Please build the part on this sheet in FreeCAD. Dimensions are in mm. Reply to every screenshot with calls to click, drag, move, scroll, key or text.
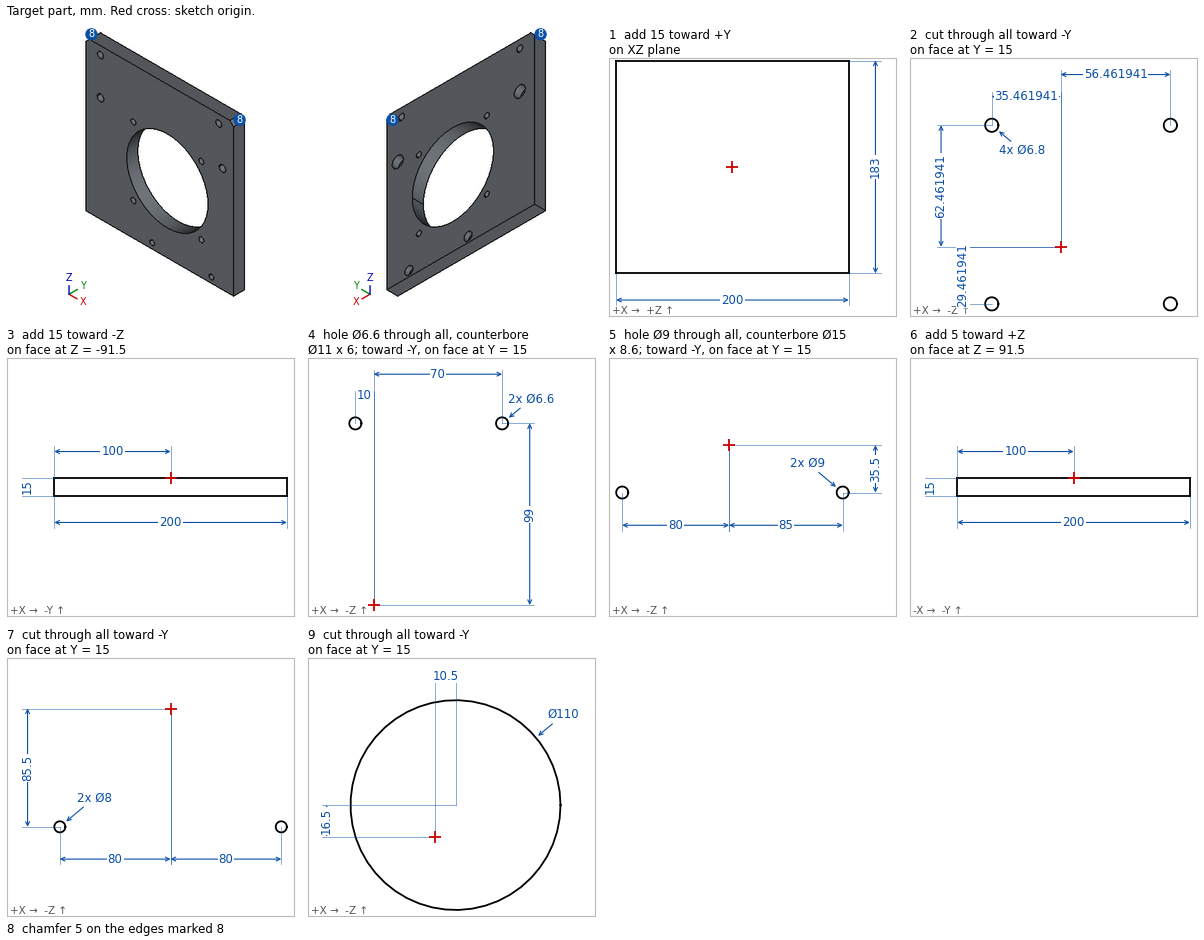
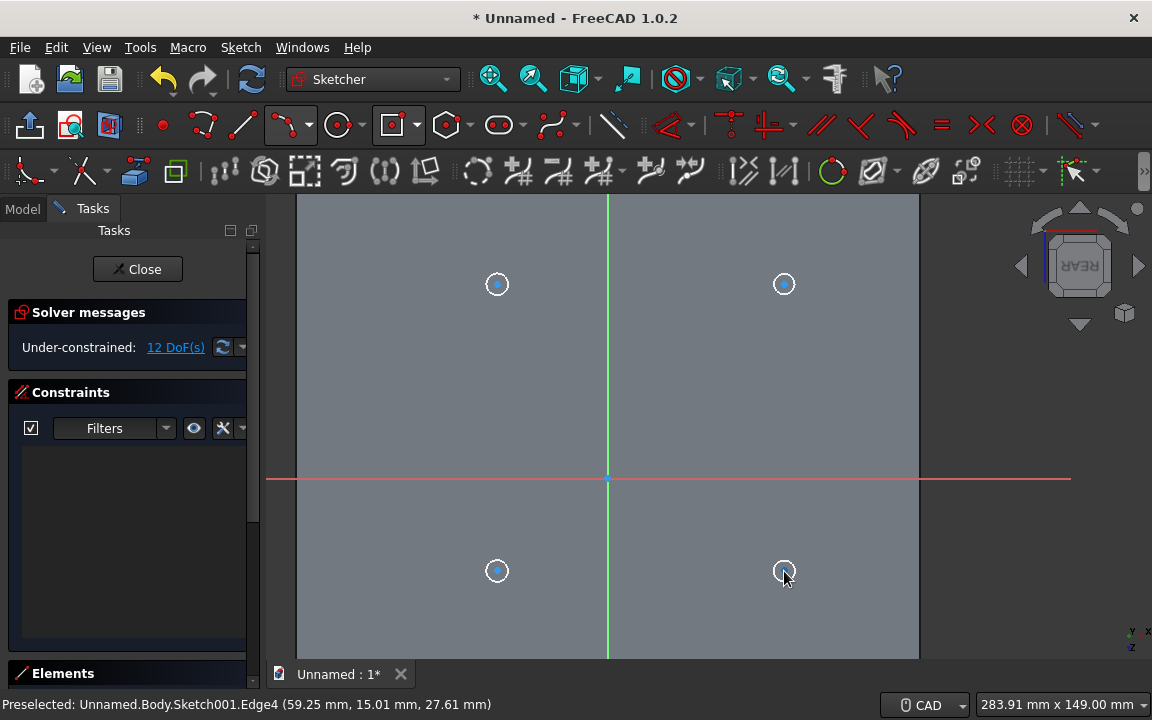
scroll(505, 277, up, 2)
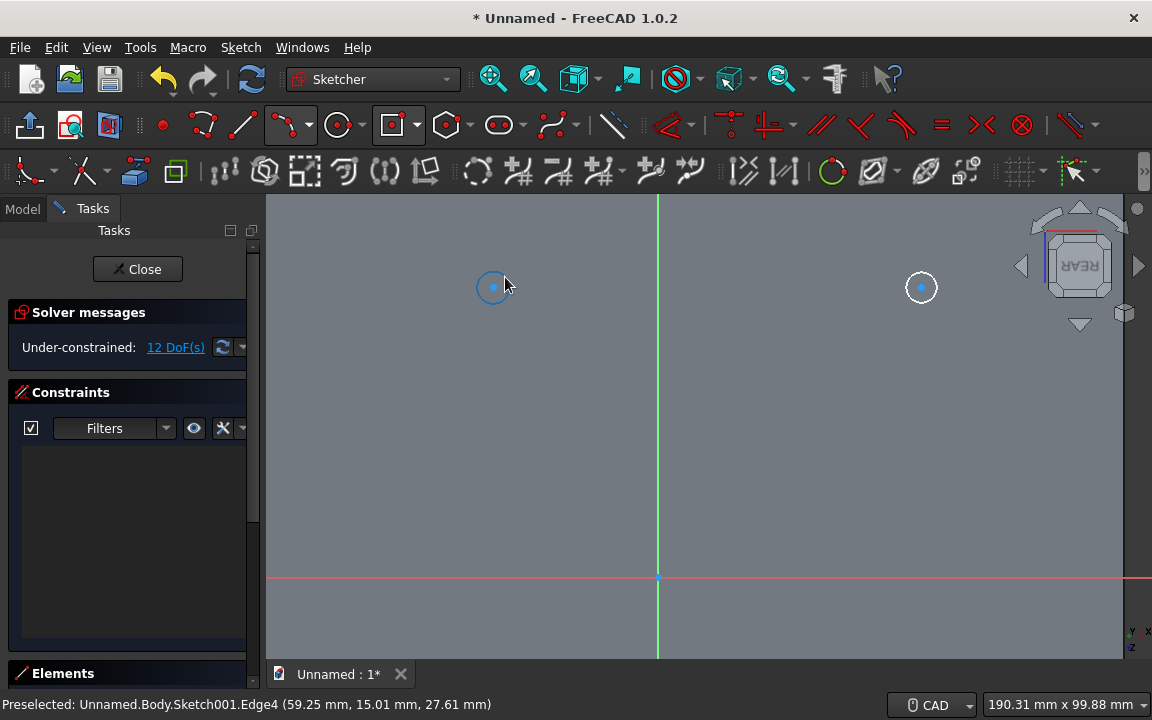
click(505, 276)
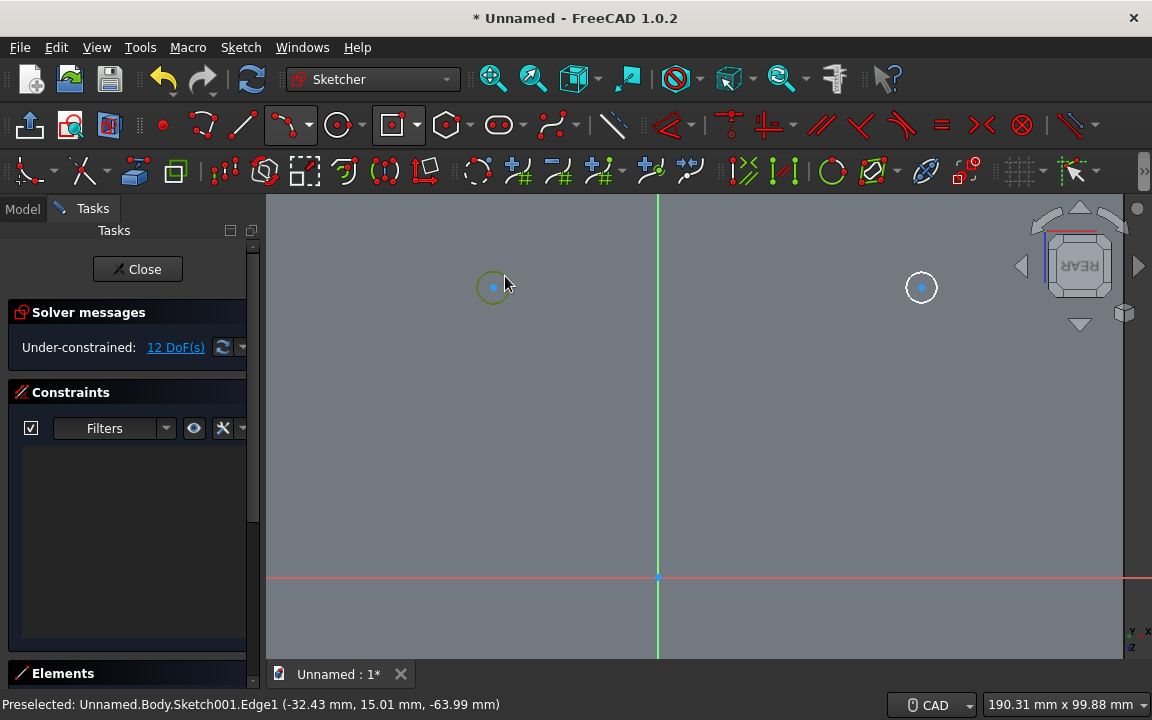
click(932, 277)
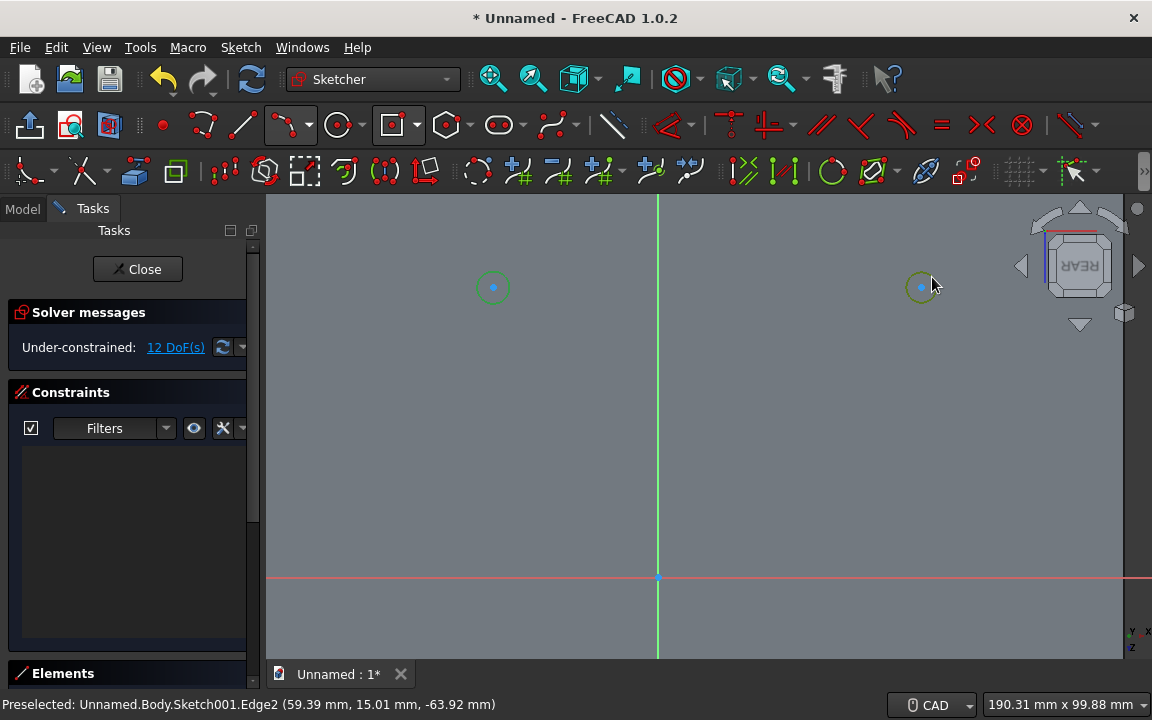
scroll(505, 275, down, 2)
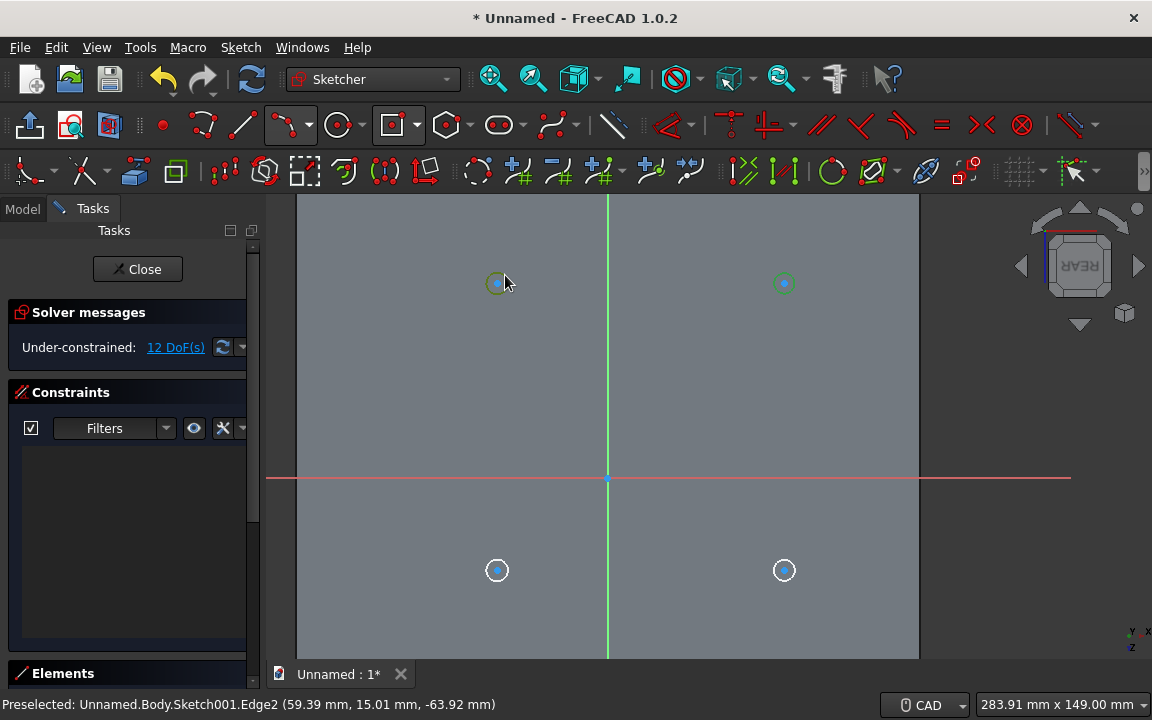
scroll(505, 563, up, 2)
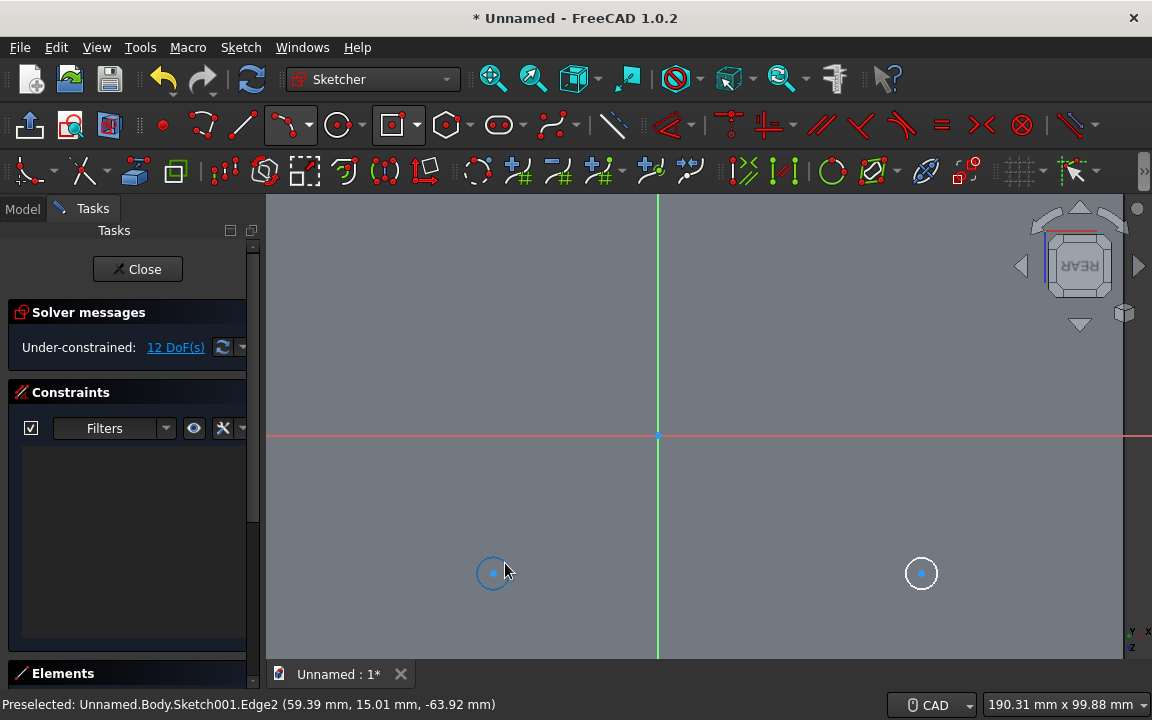
click(505, 562)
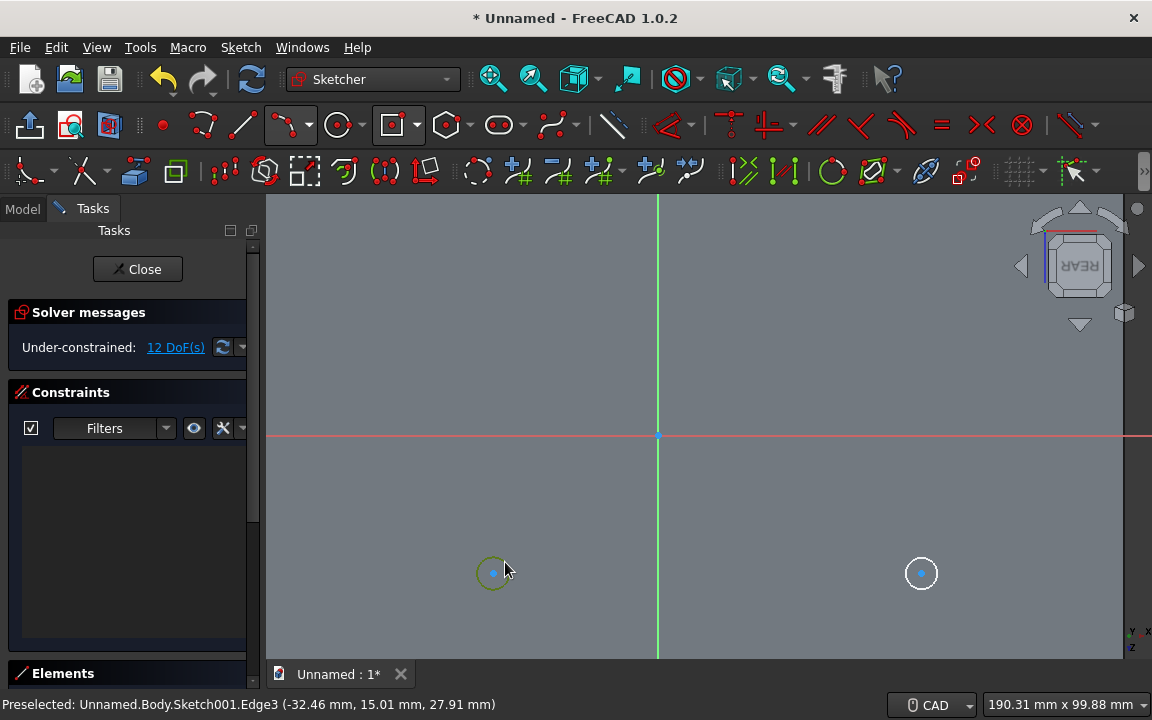
click(933, 562)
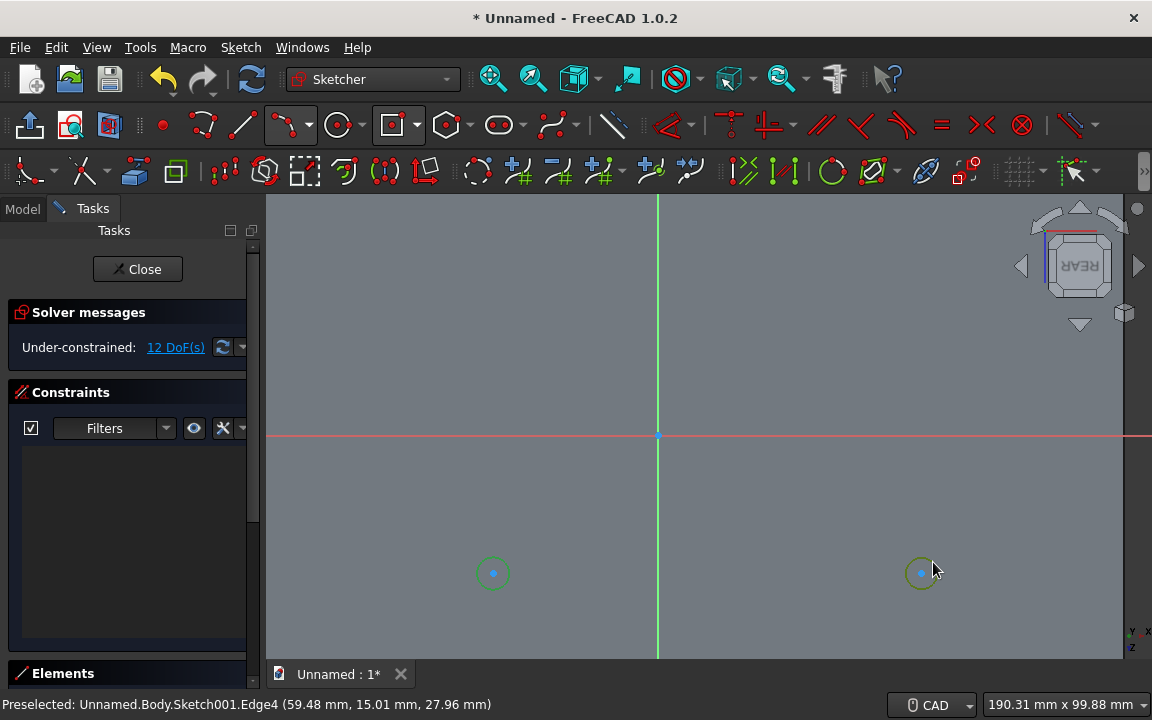
click(942, 126)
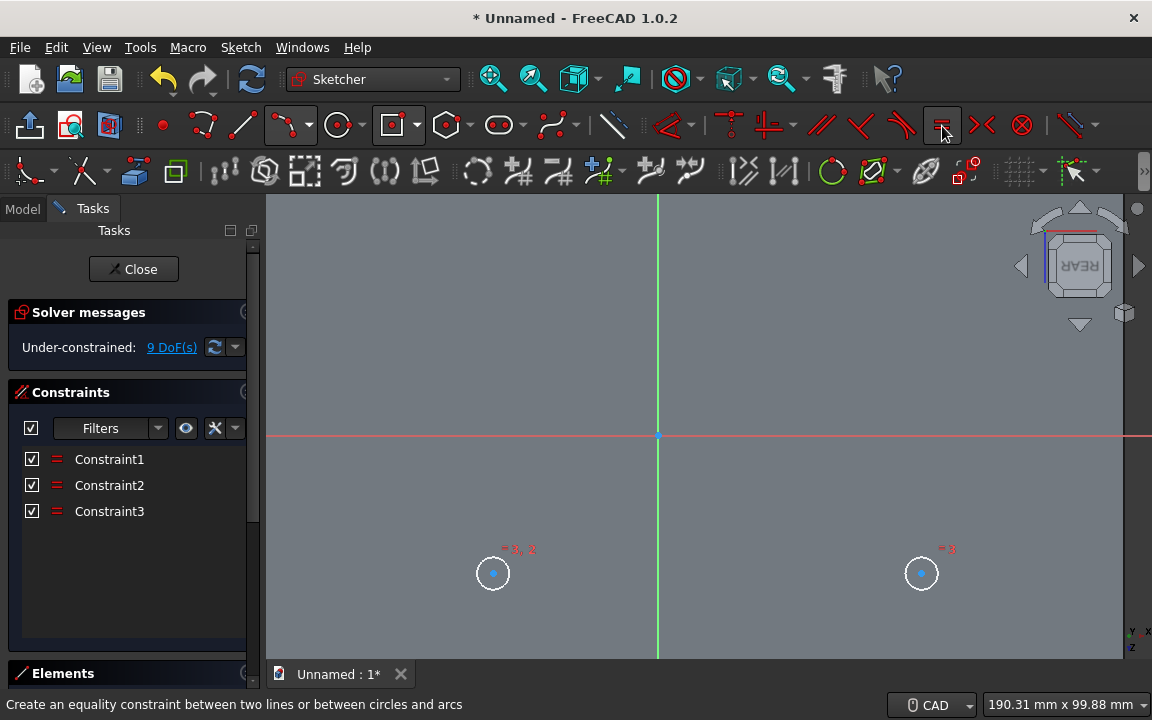
scroll(505, 564, down, 2)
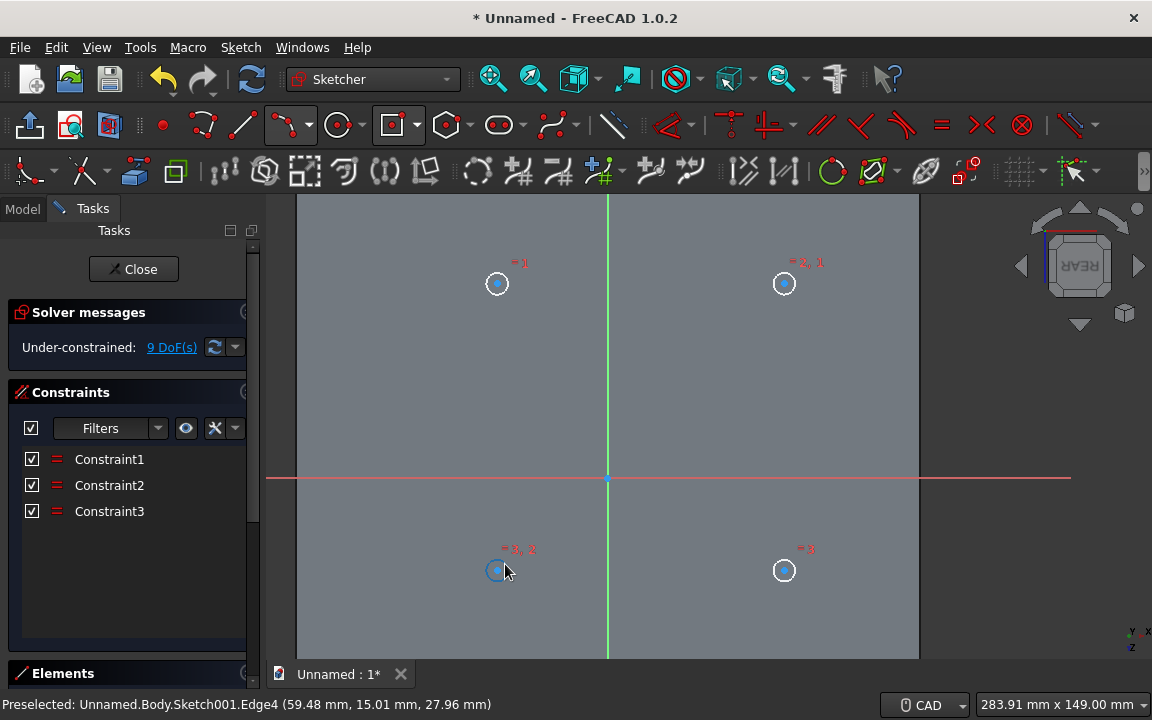
click(497, 284)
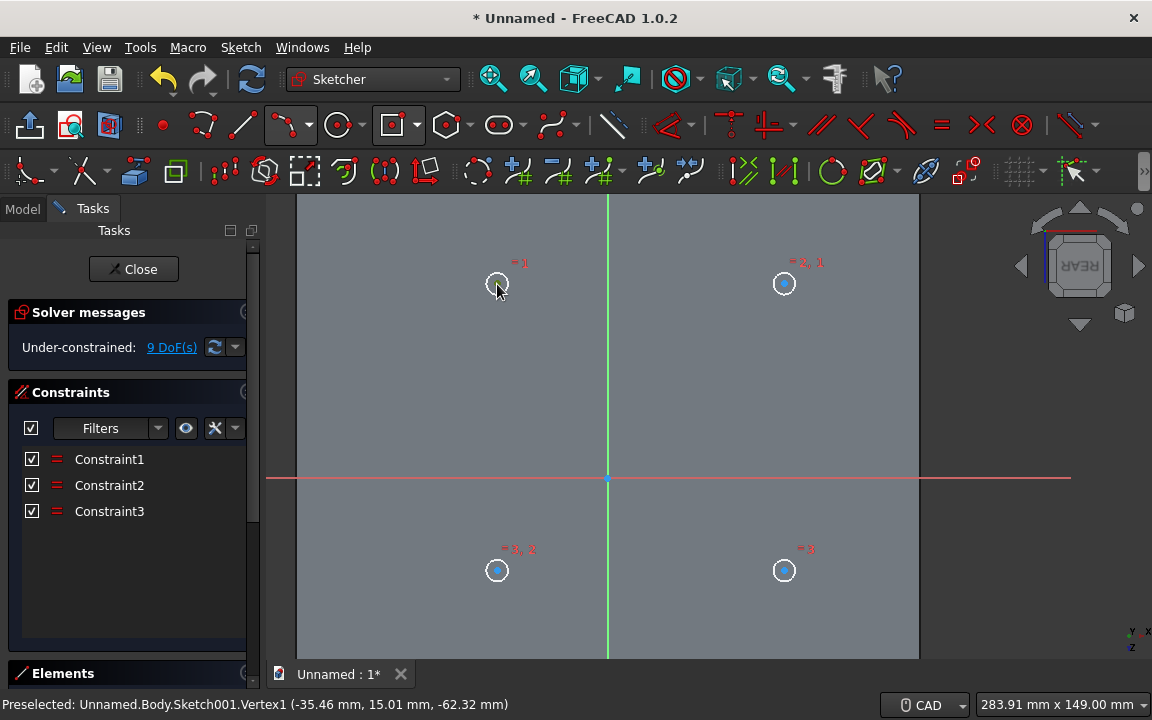
click(784, 284)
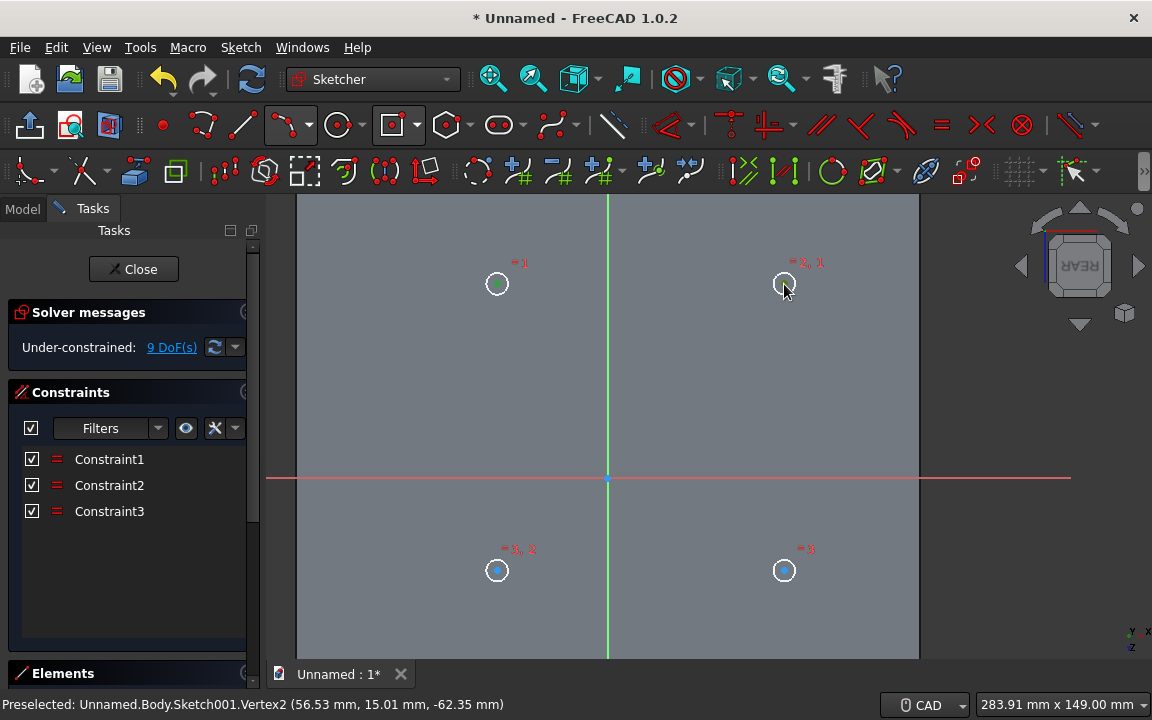
key(h)